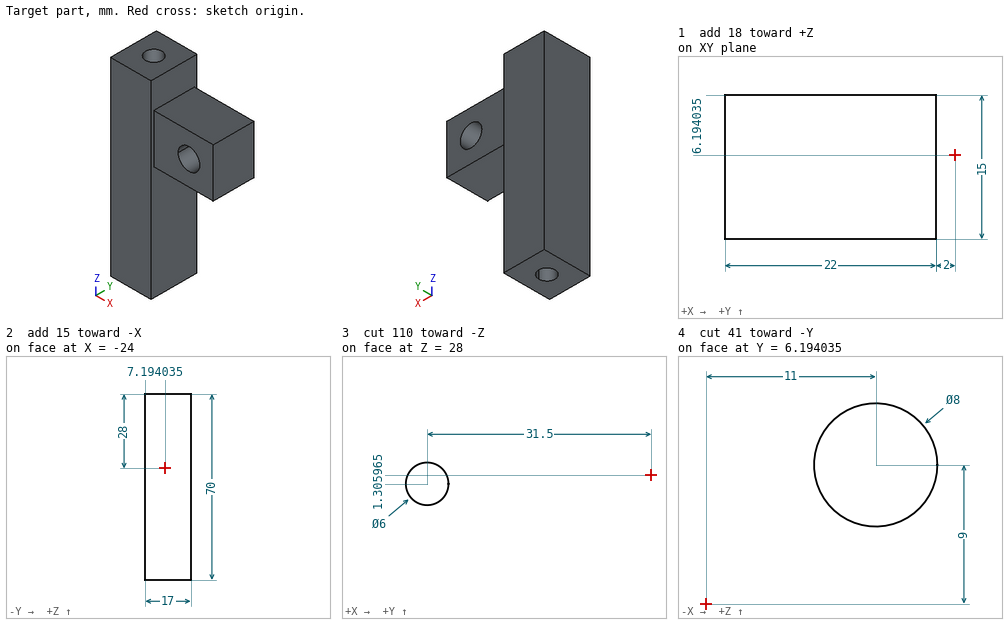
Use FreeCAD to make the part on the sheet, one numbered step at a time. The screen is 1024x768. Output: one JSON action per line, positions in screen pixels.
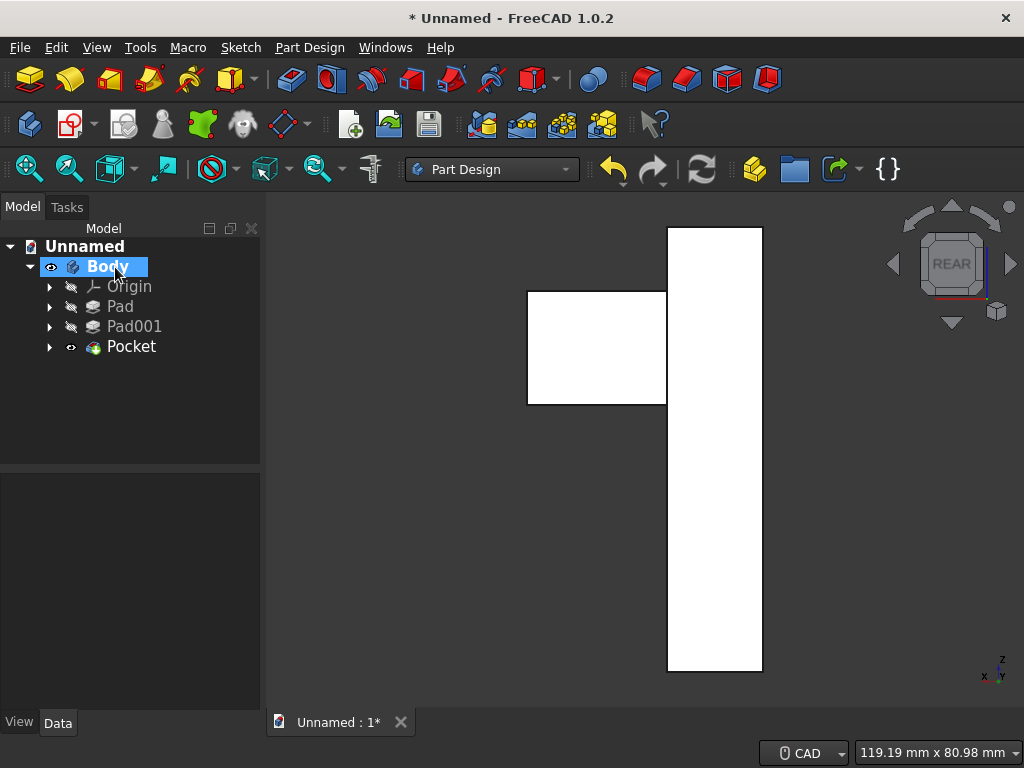
{"action": "left_click", "coordinate": [597, 347]}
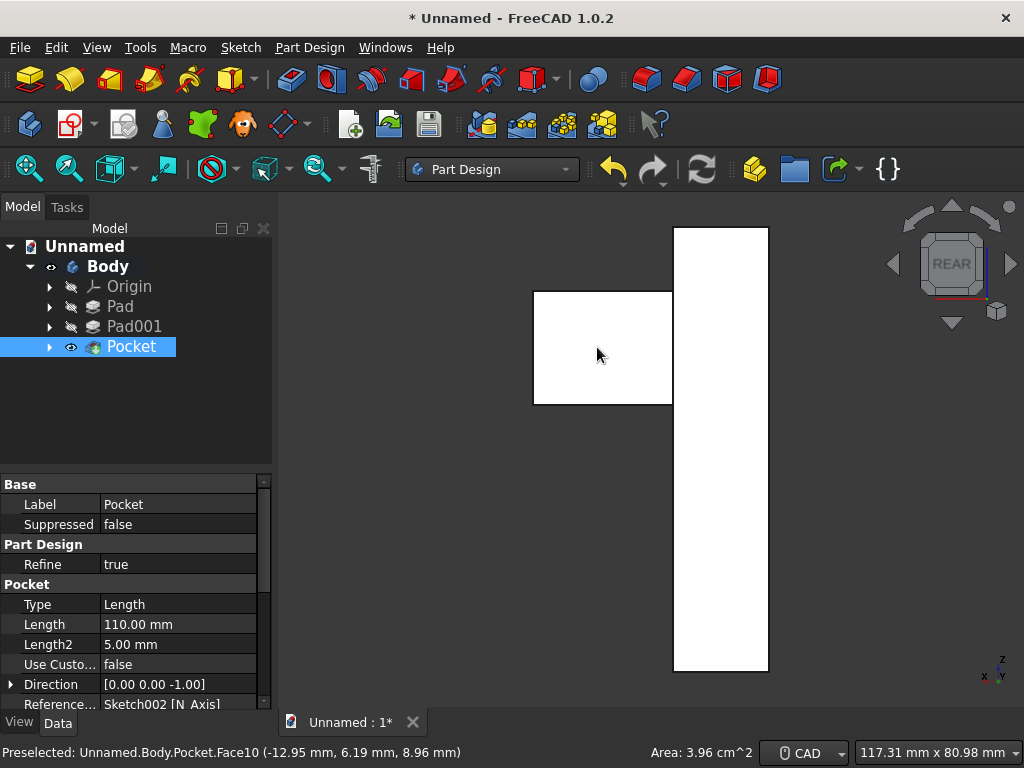
{"action": "left_click", "coordinate": [70, 124]}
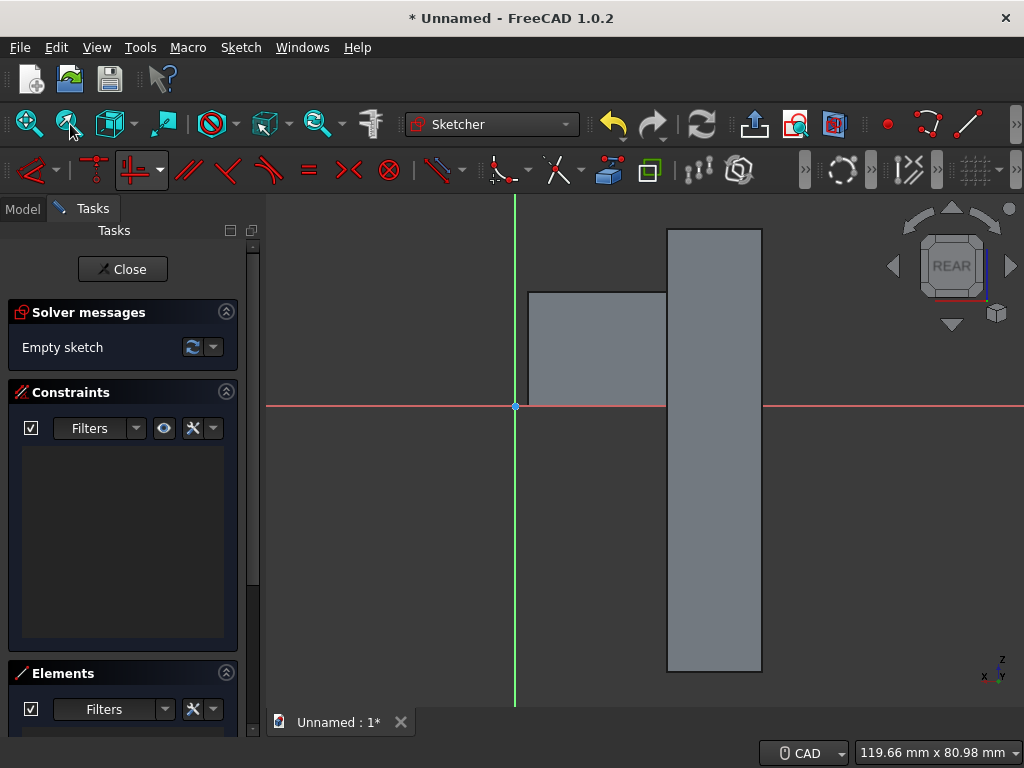
{"action": "left_click", "coordinate": [836, 124]}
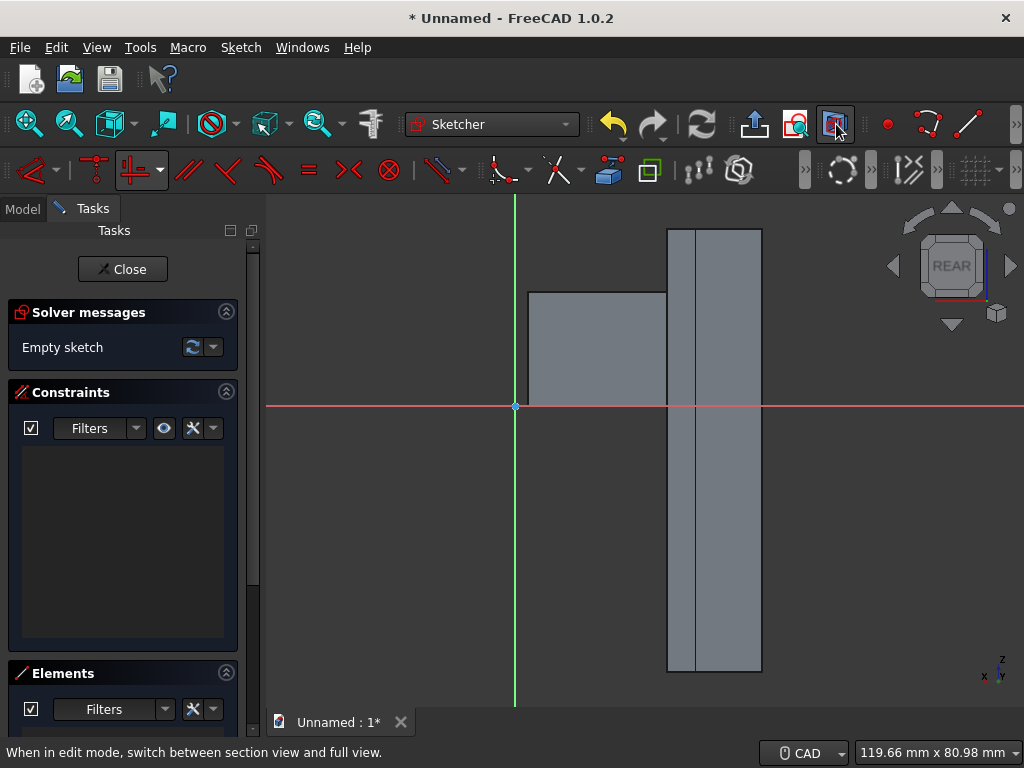
{"action": "scroll", "coordinate": [558, 337], "scroll_direction": "up", "scroll_amount": 7}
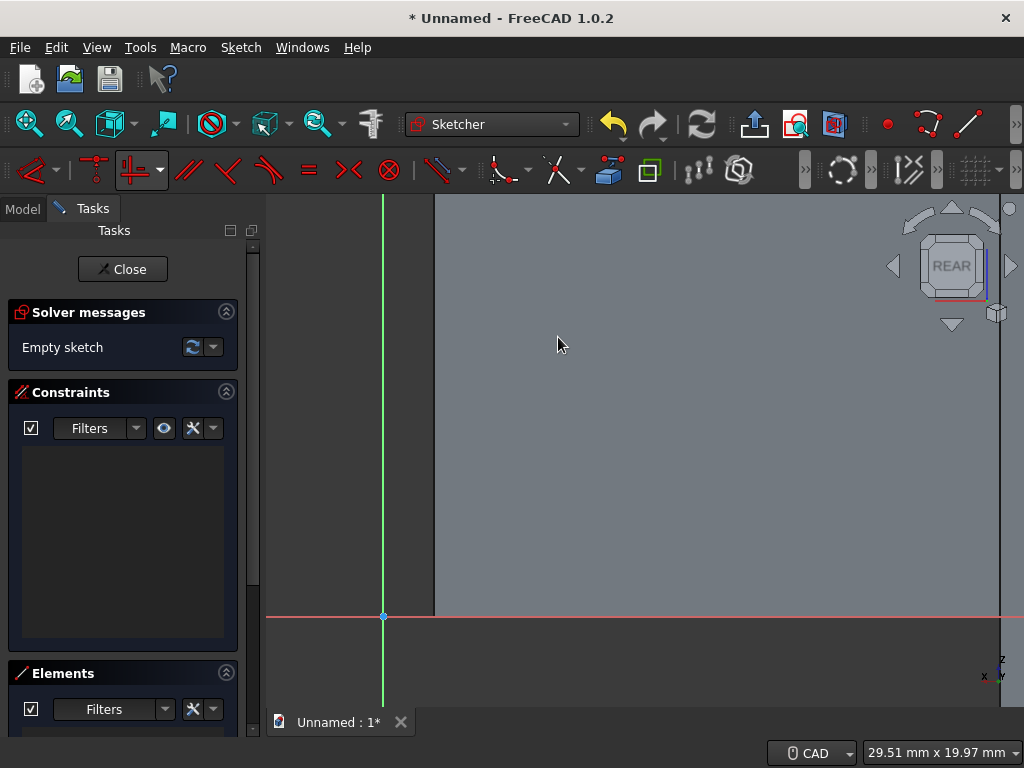
{"action": "key", "text": "g c"}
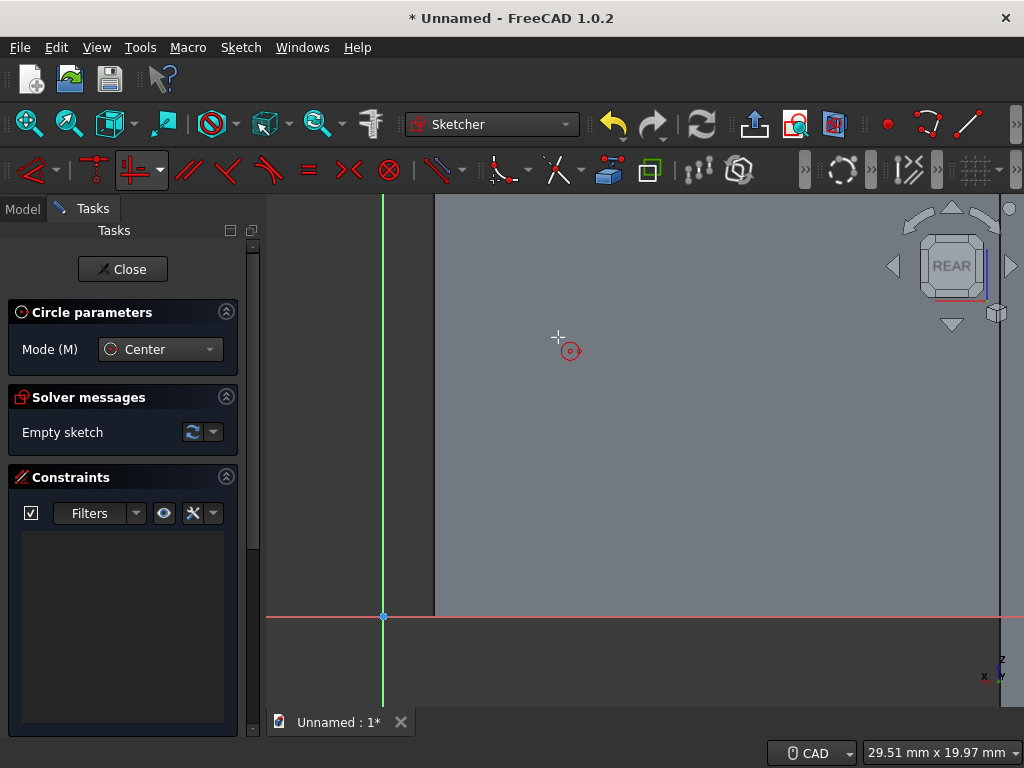
{"action": "left_click", "coordinate": [666, 385]}
{"action": "mouse_move", "coordinate": [738, 313]}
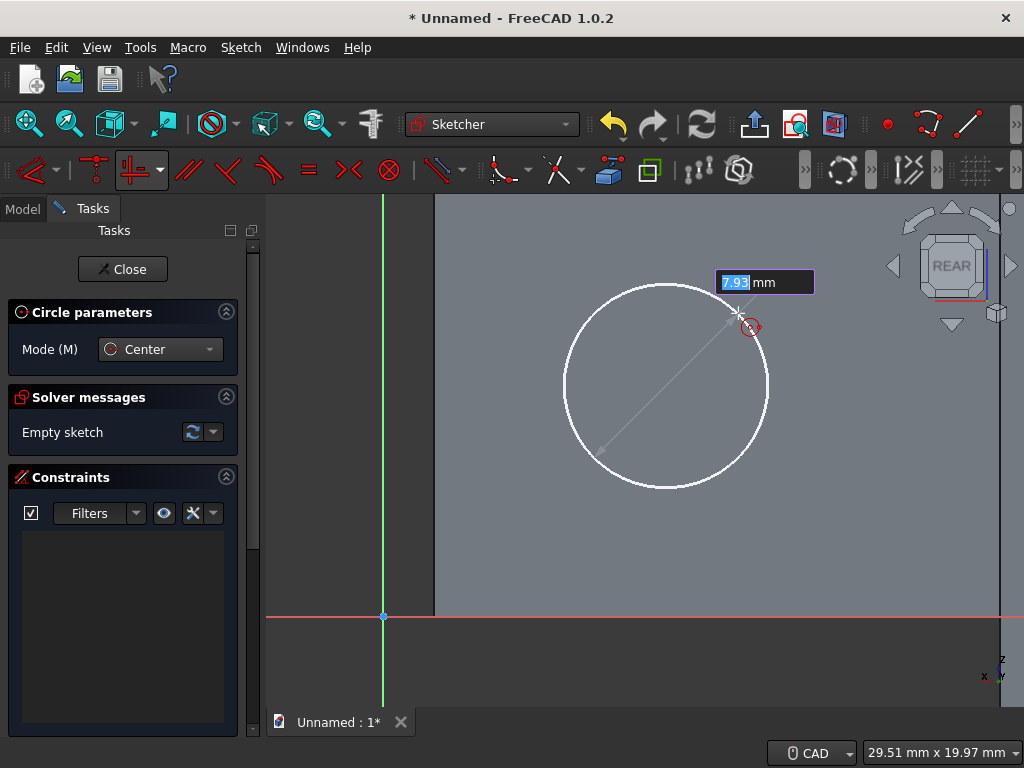
{"action": "type", "text": "8"}
{"action": "key", "text": "Return"}
{"action": "key", "text": "Escape"}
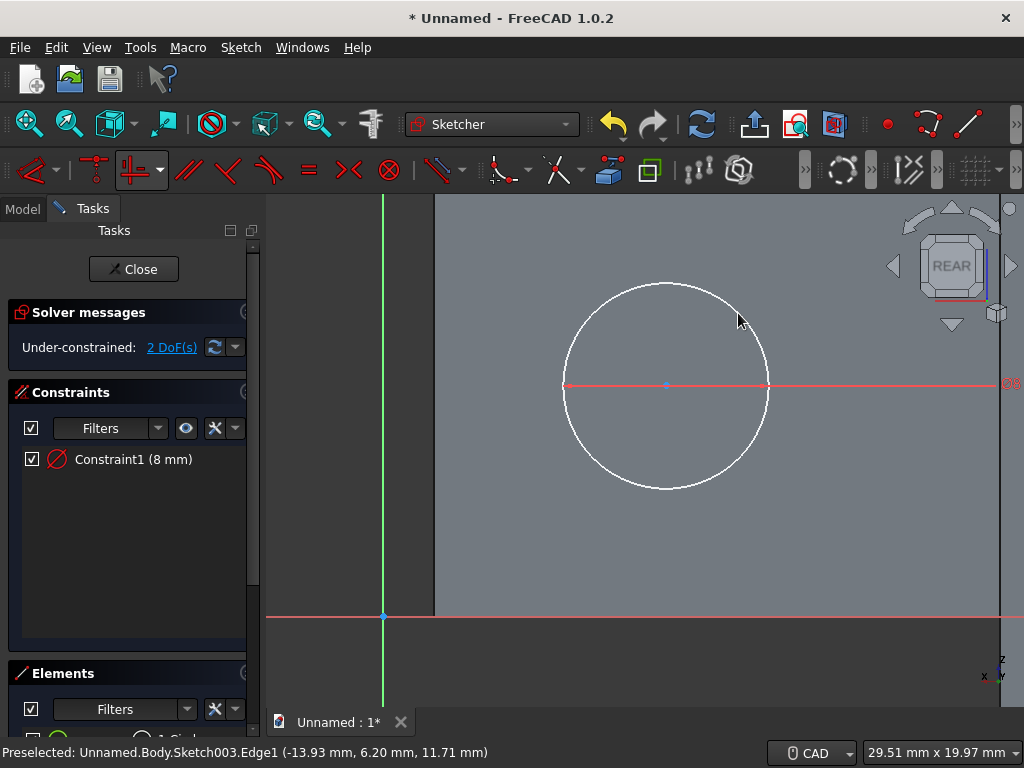
{"action": "key", "text": "d"}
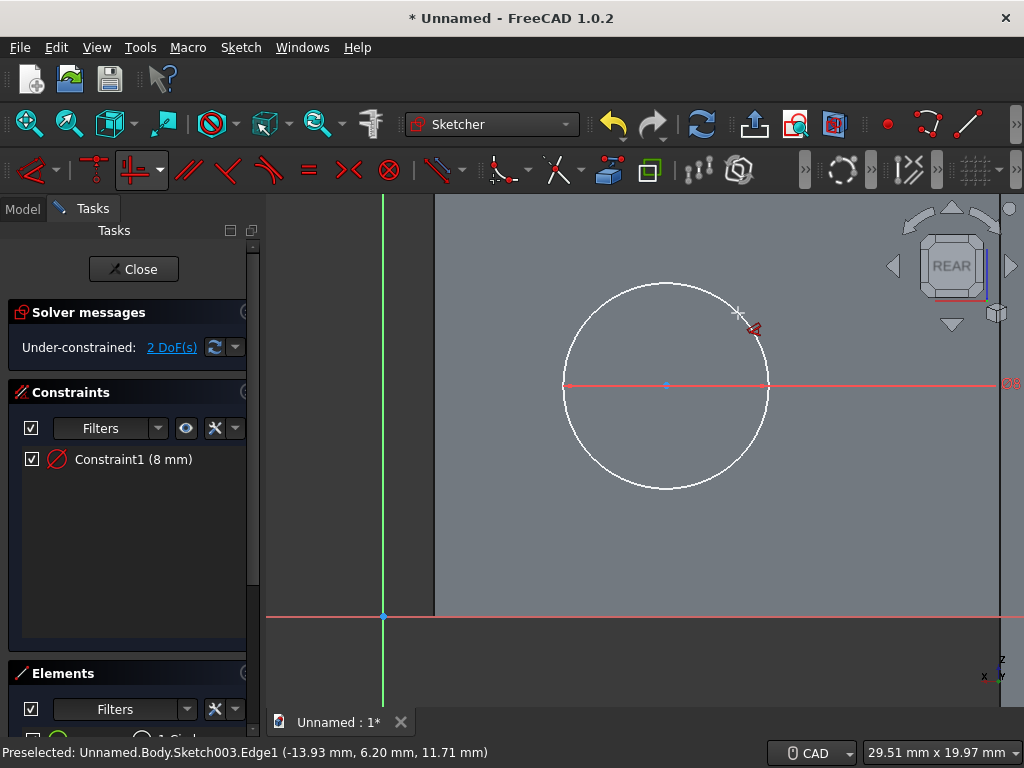
{"action": "left_click", "coordinate": [666, 386]}
{"action": "left_click", "coordinate": [349, 501]}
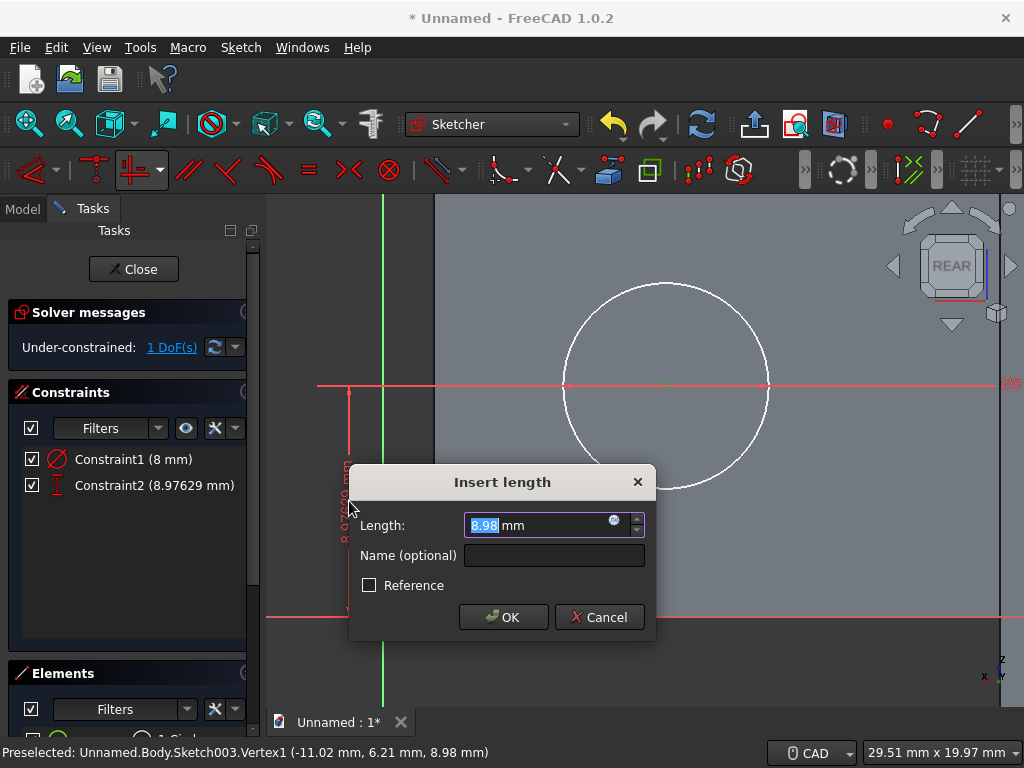
{"action": "type", "text": "9"}
{"action": "key", "text": "Return"}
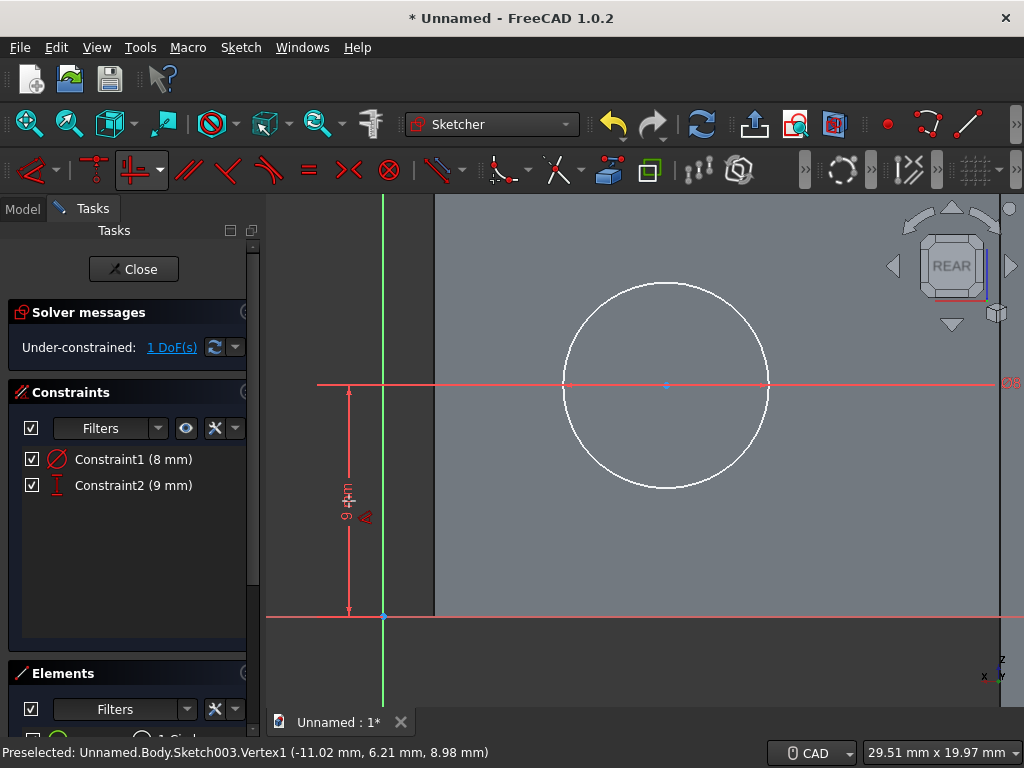
{"action": "left_click", "coordinate": [666, 385]}
{"action": "left_click", "coordinate": [525, 651]}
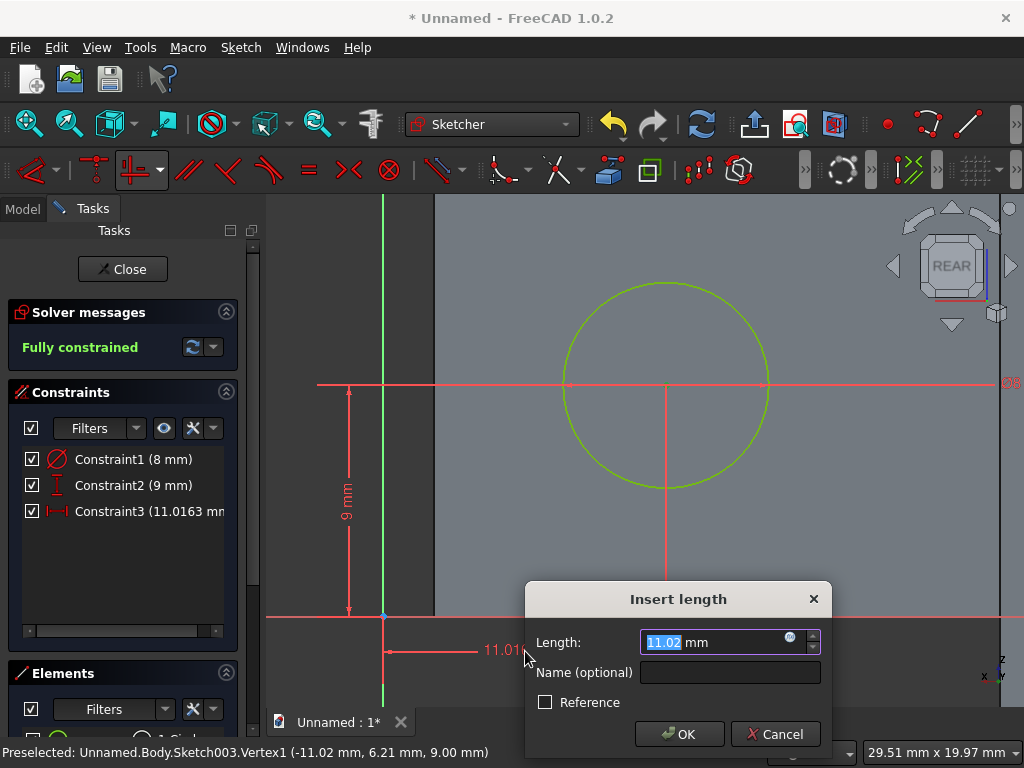
{"action": "type", "text": "11"}
{"action": "key", "text": "Return"}
{"action": "key", "text": "Escape"}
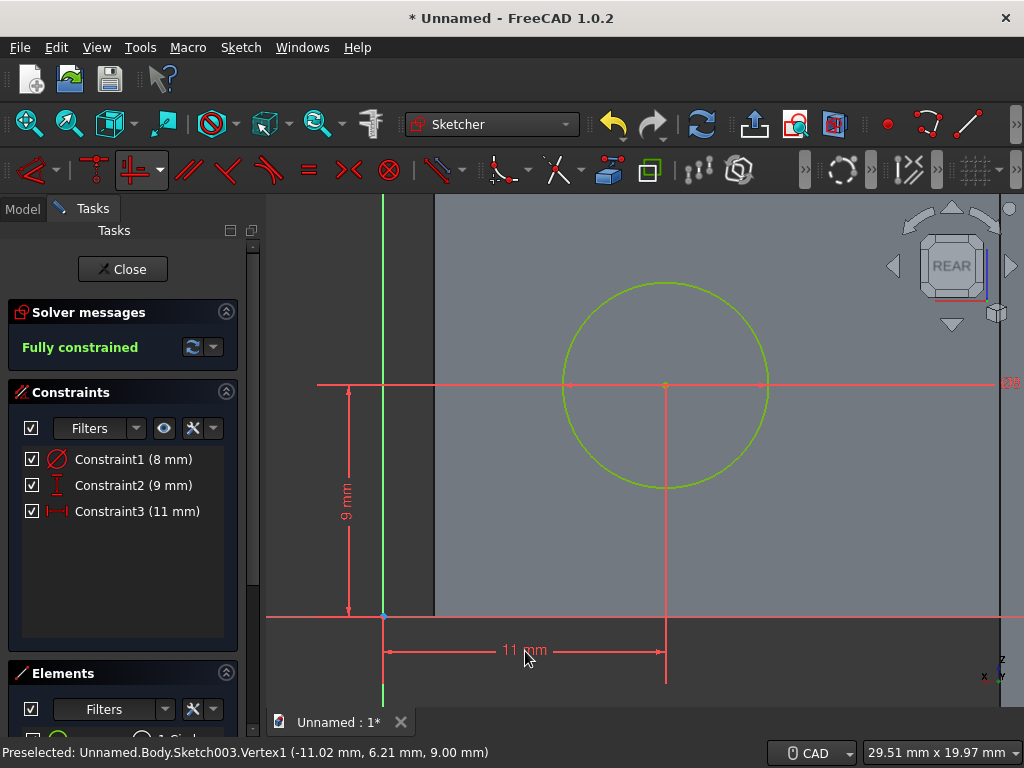
{"action": "left_click", "coordinate": [123, 269]}